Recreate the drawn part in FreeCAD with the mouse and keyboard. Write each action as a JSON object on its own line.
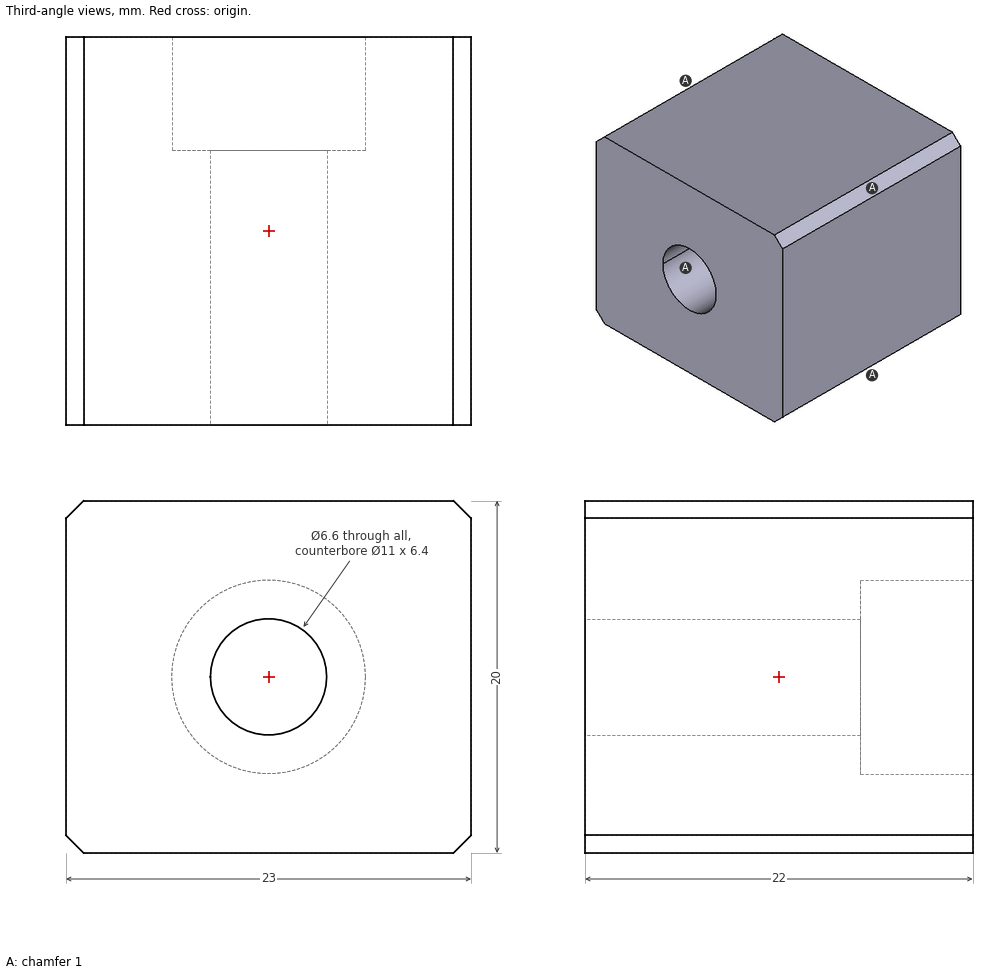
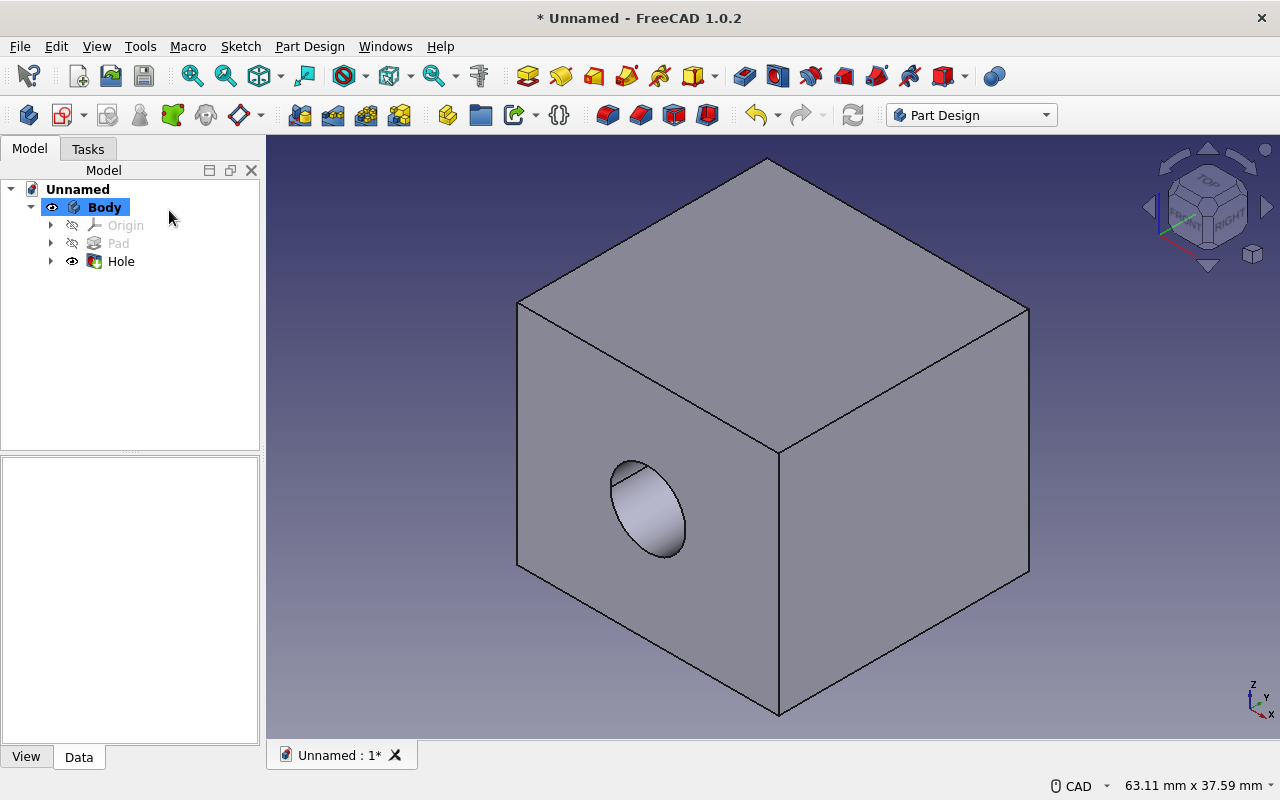
{"action": "left_click", "coordinate": [904, 380]}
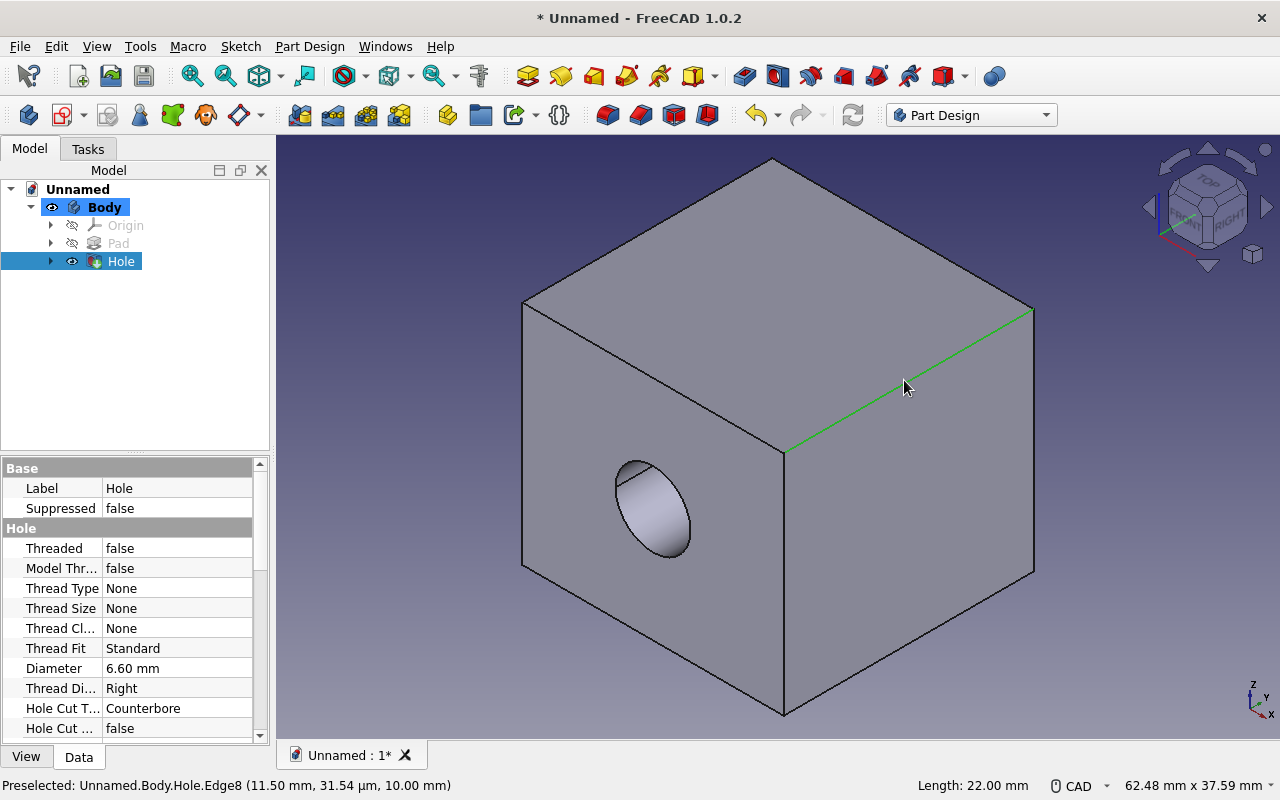
{"action": "key", "text": "2"}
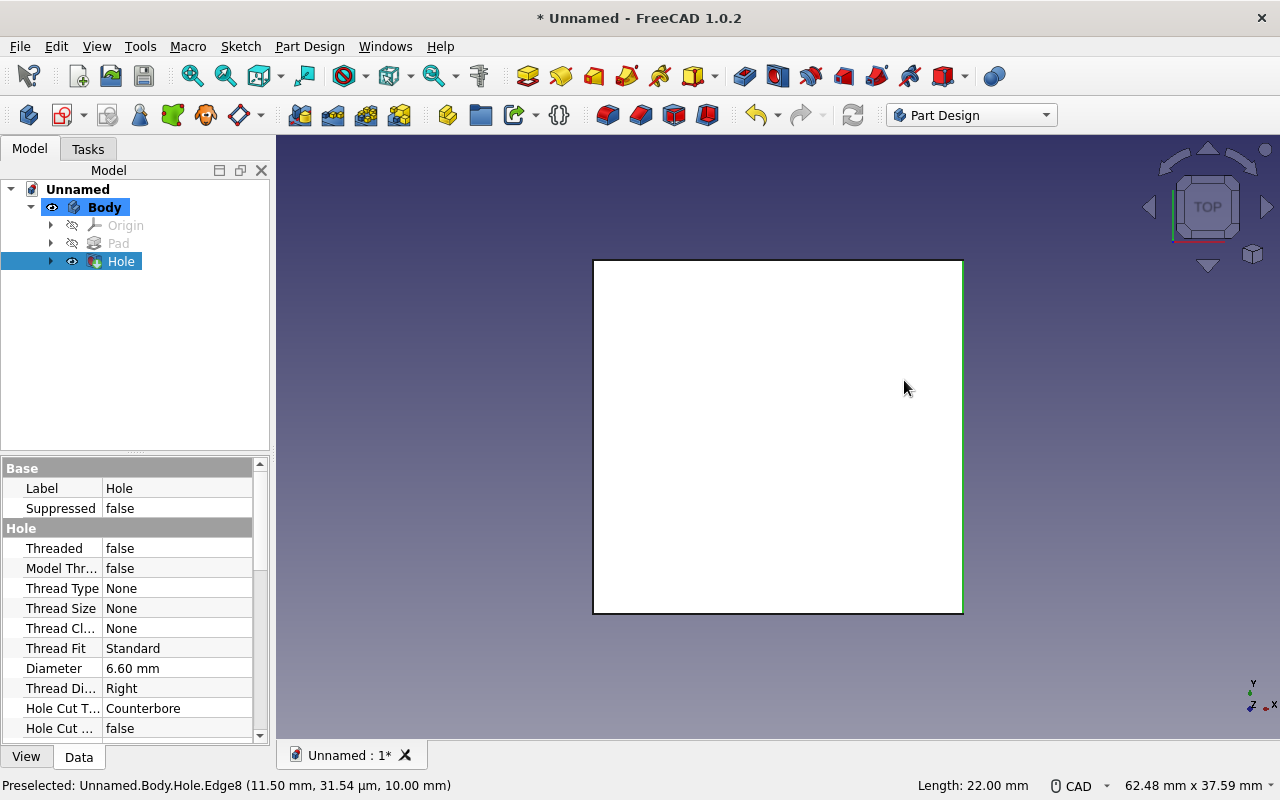
{"action": "left_click", "coordinate": [593, 436], "text": "ctrl"}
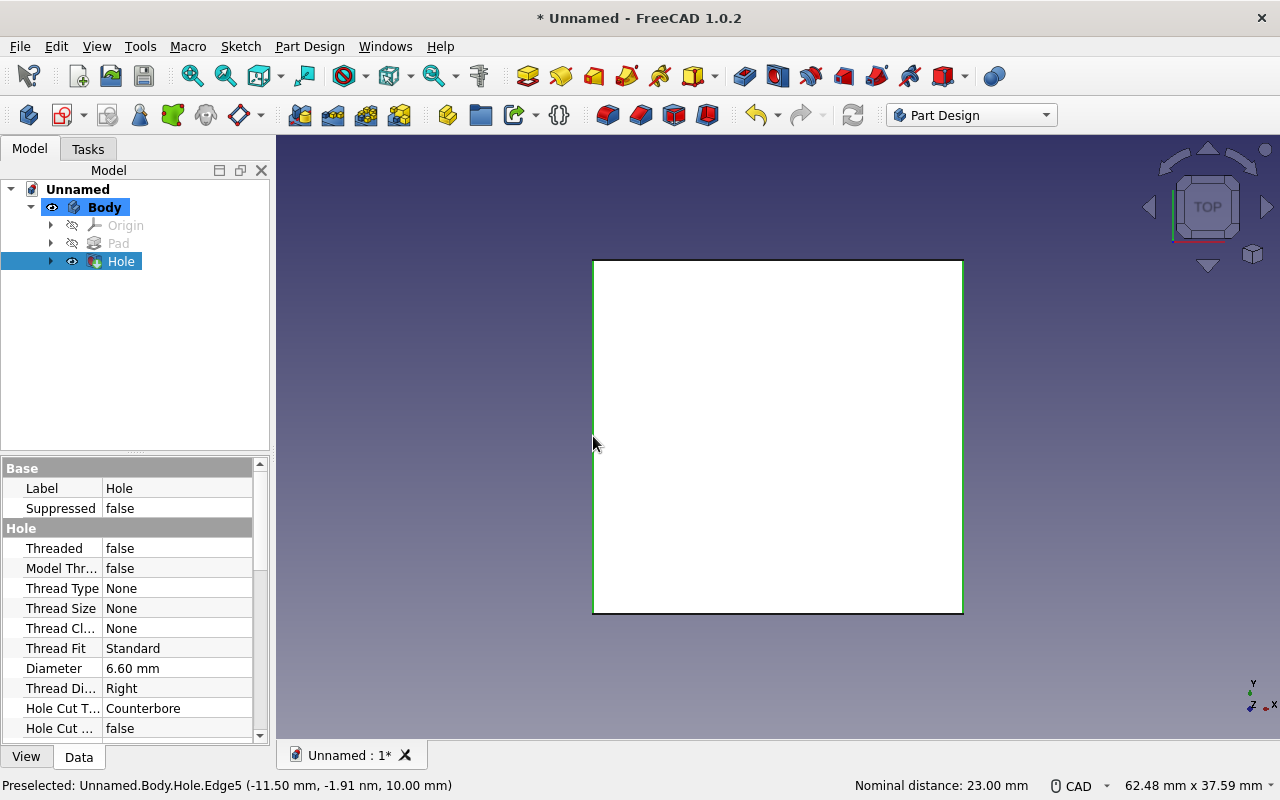
{"action": "key", "text": "1"}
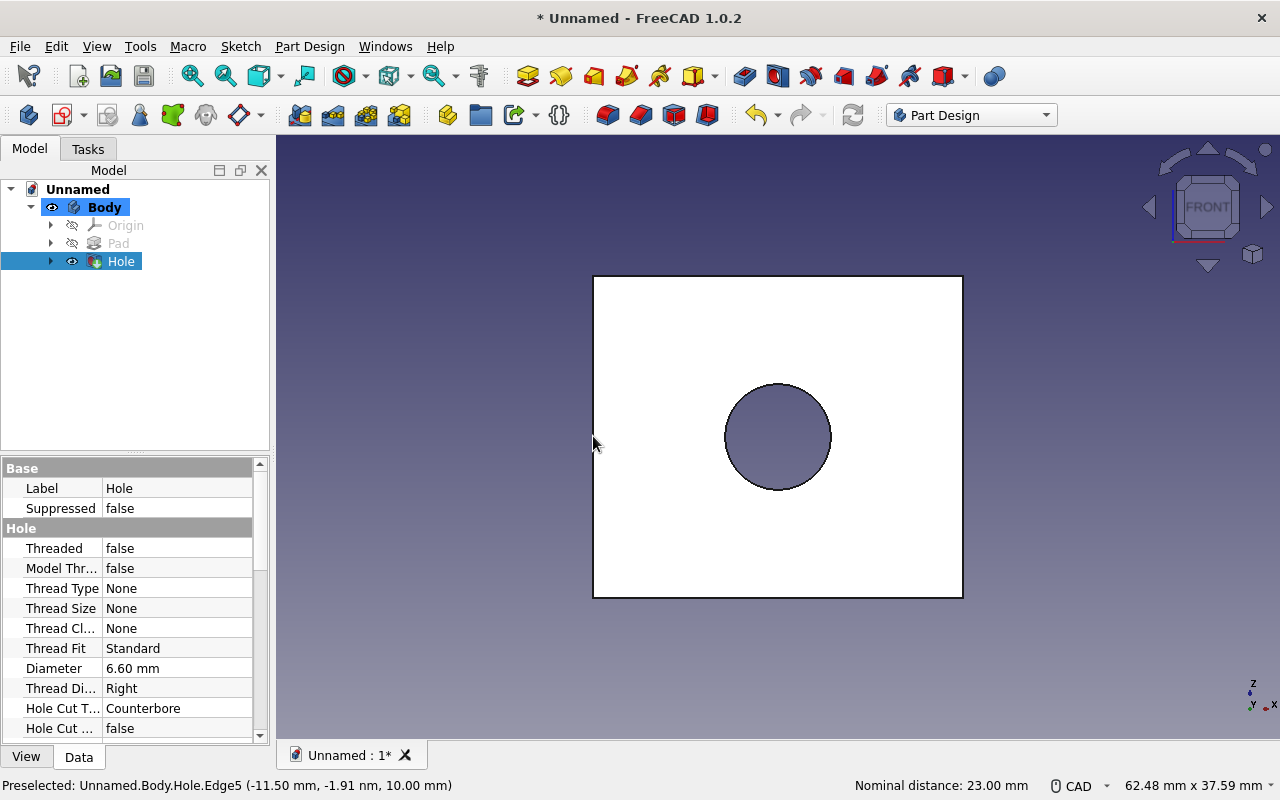
{"action": "key", "text": "3"}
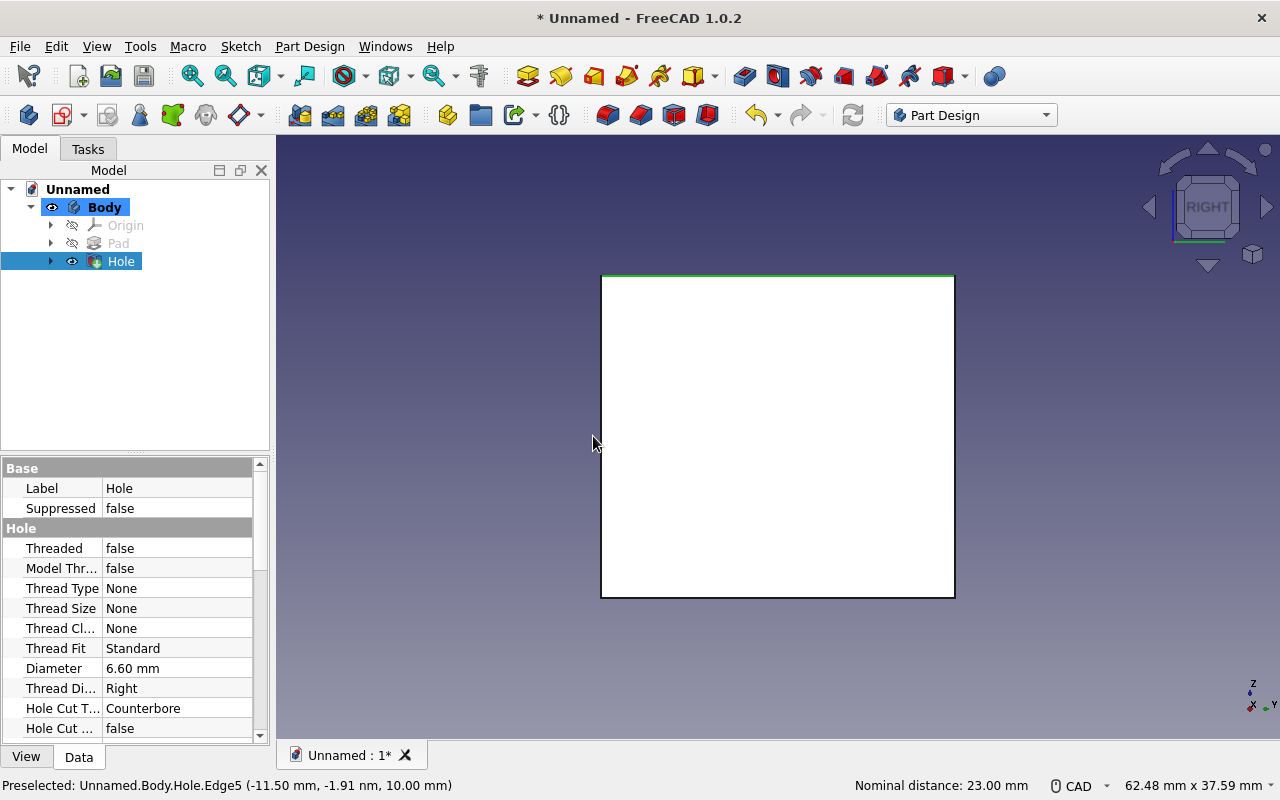
{"action": "left_click", "coordinate": [778, 597], "text": "ctrl"}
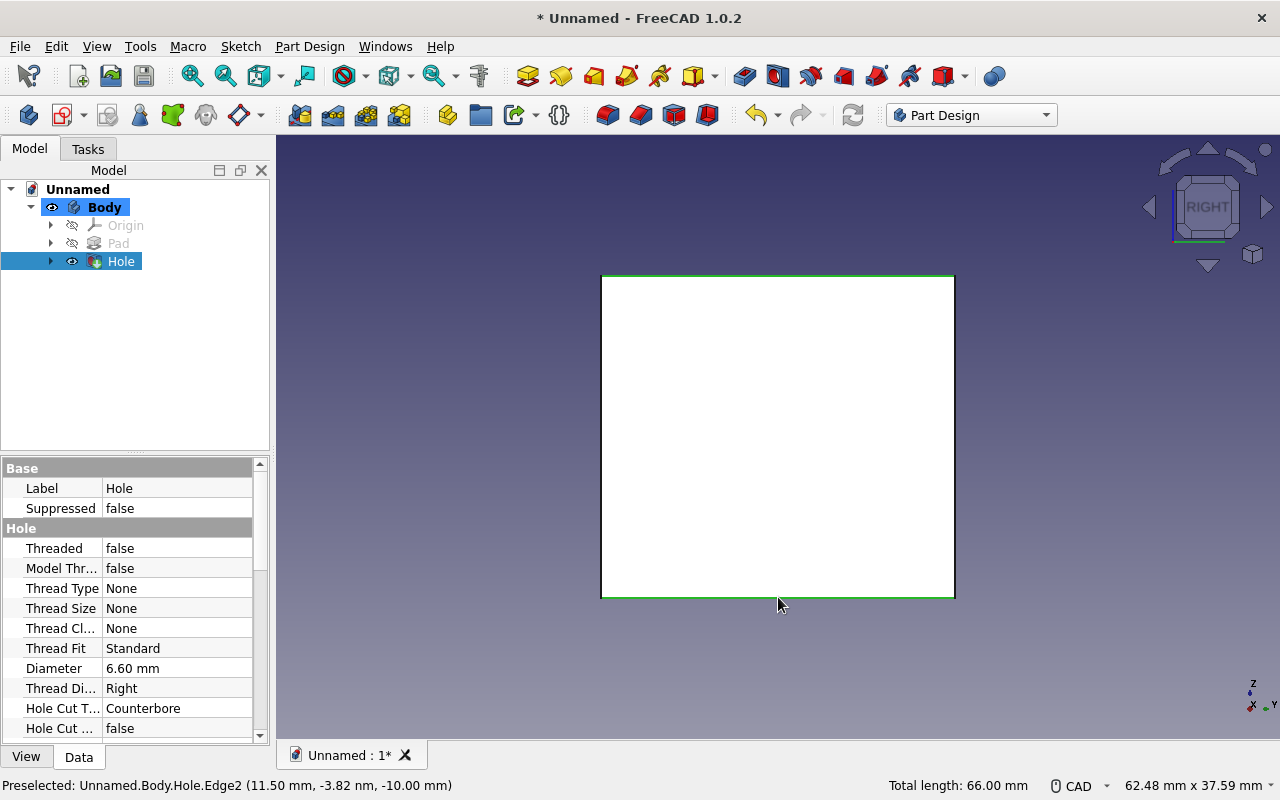
{"action": "key", "text": "5"}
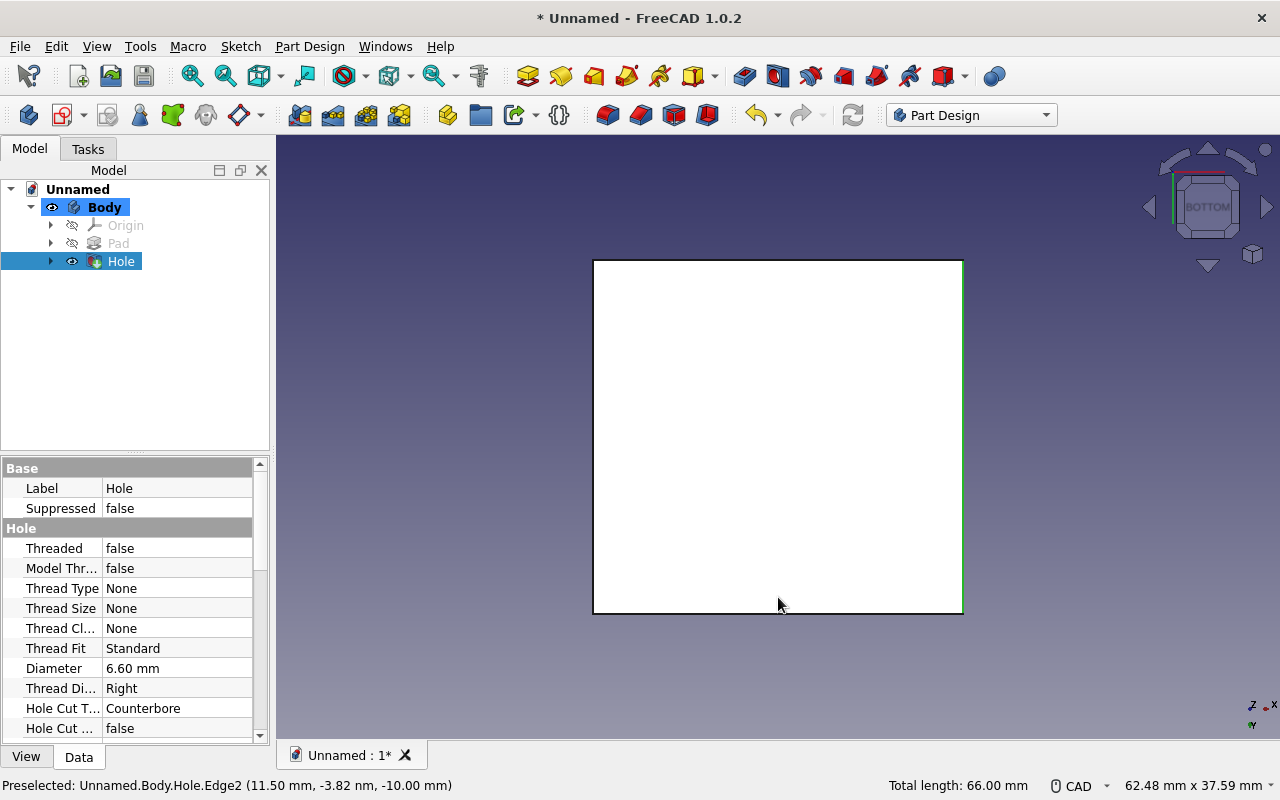
{"action": "left_click", "coordinate": [593, 436], "text": "ctrl"}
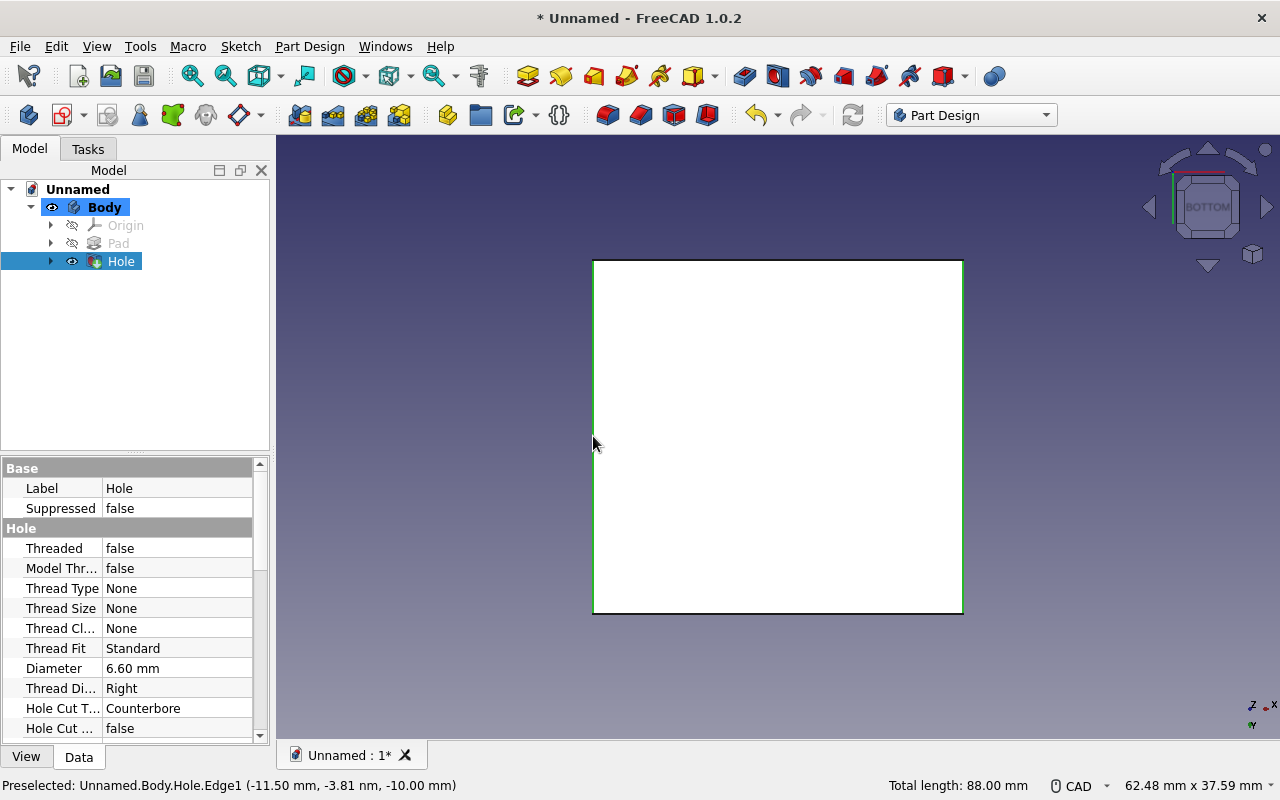
{"action": "left_click", "coordinate": [641, 116]}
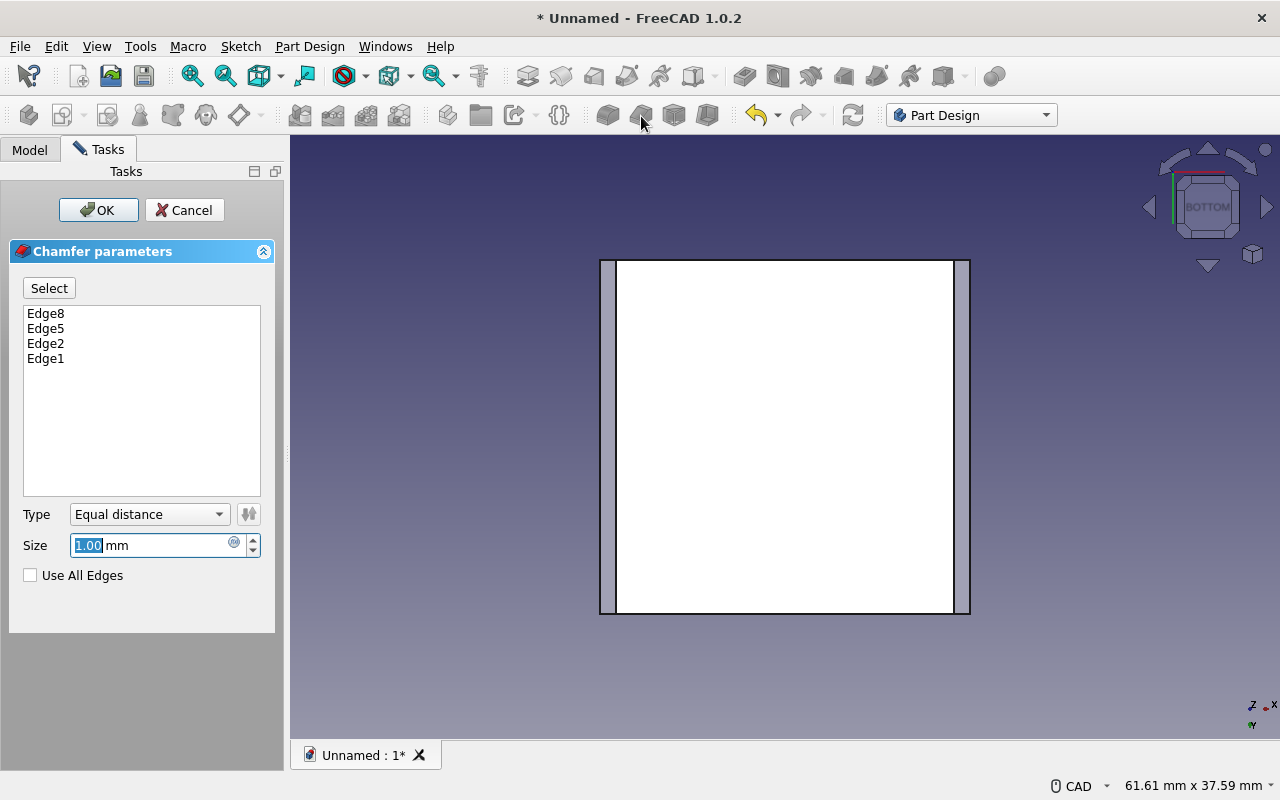
{"action": "type", "text": "1"}
{"action": "key", "text": "Tab"}